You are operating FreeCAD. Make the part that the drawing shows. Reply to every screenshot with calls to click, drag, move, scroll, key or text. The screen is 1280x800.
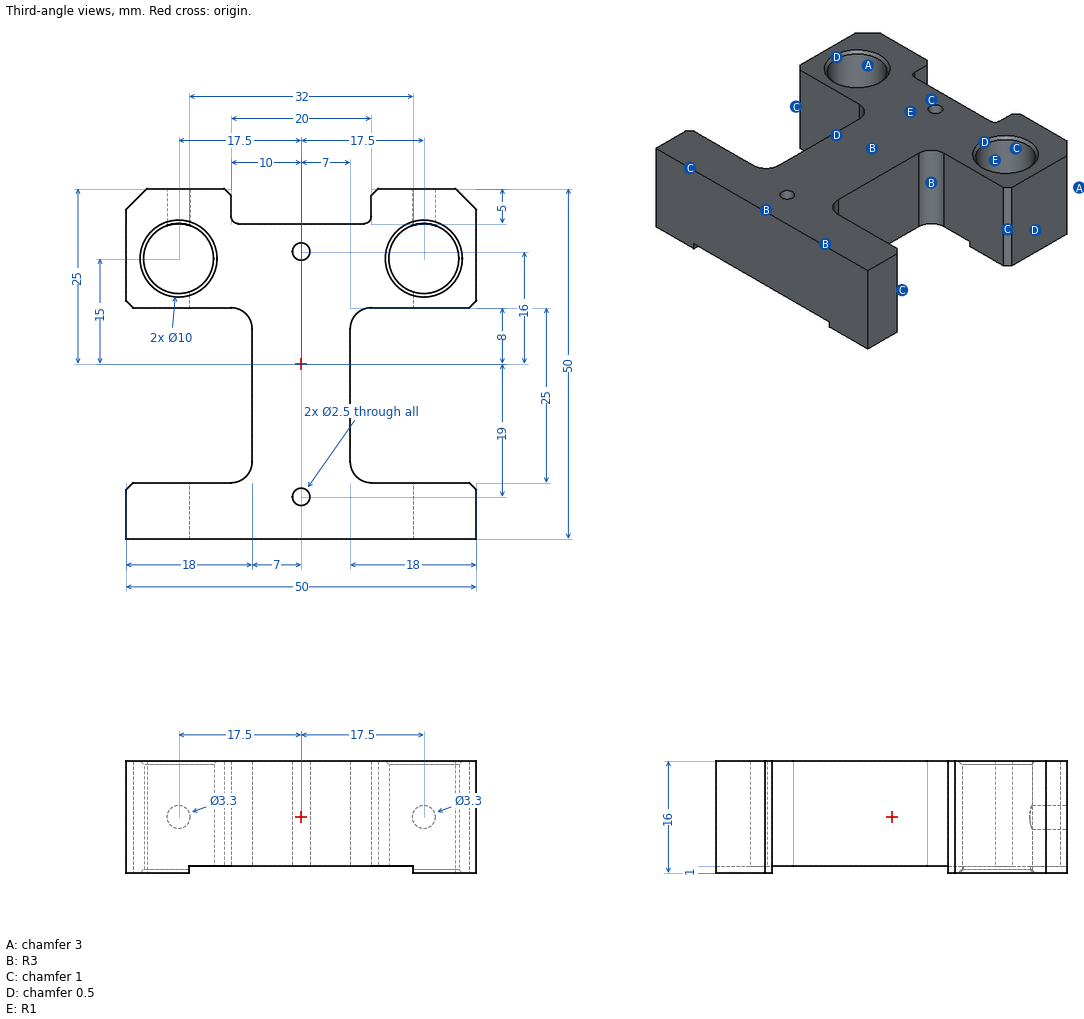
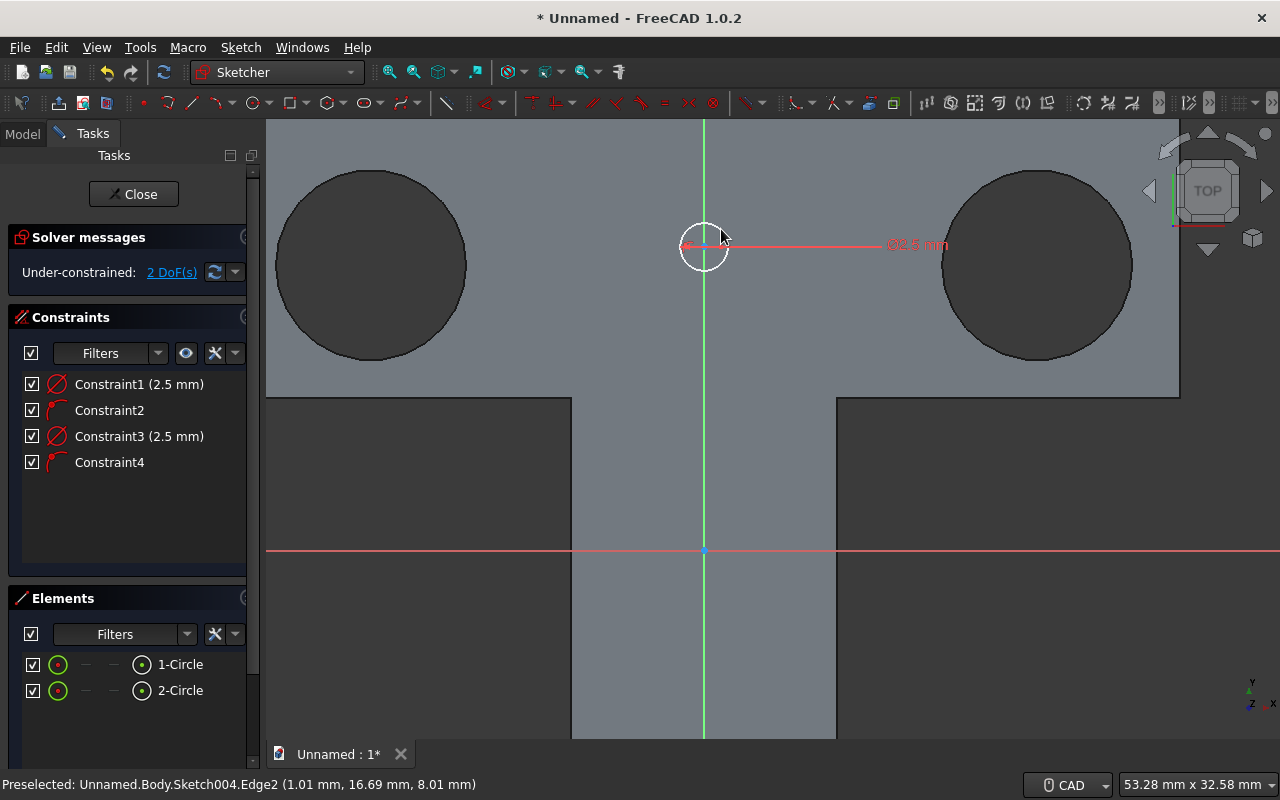
key(d)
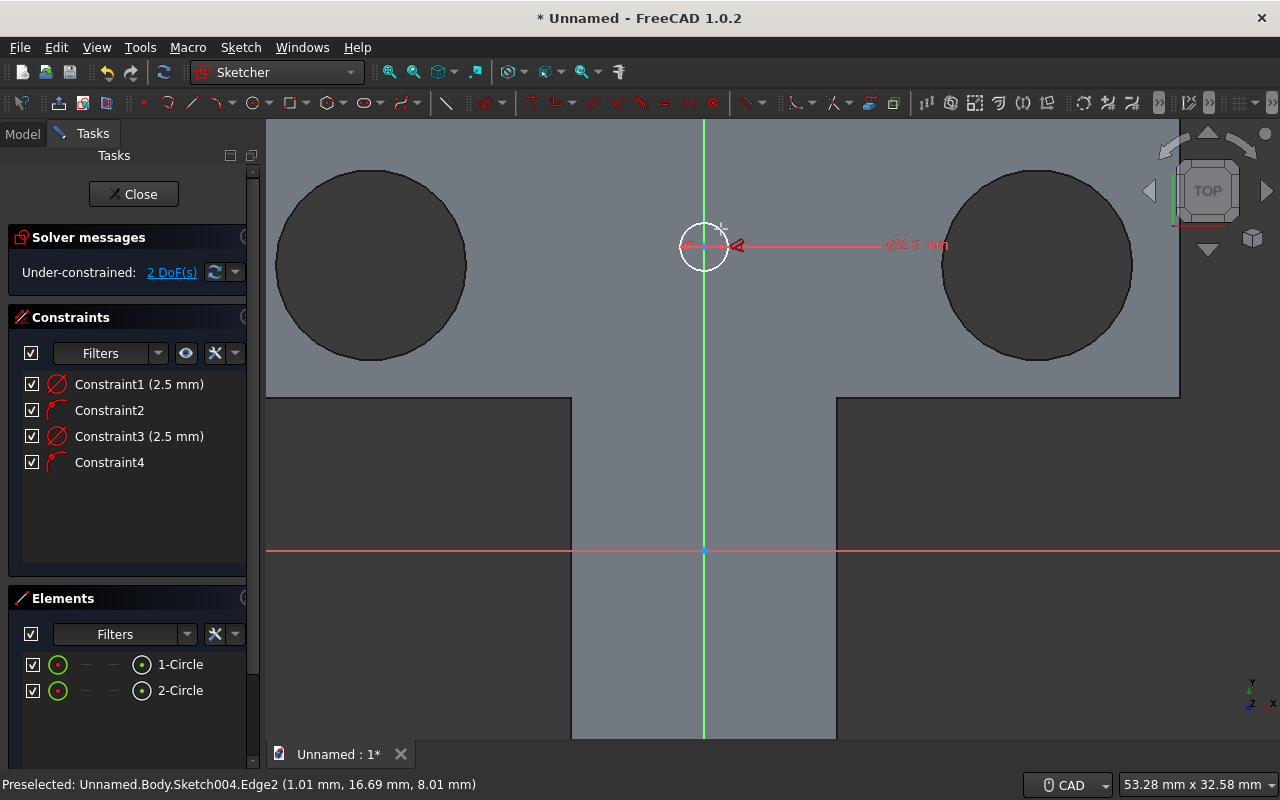
scroll(705, 246, down, 3)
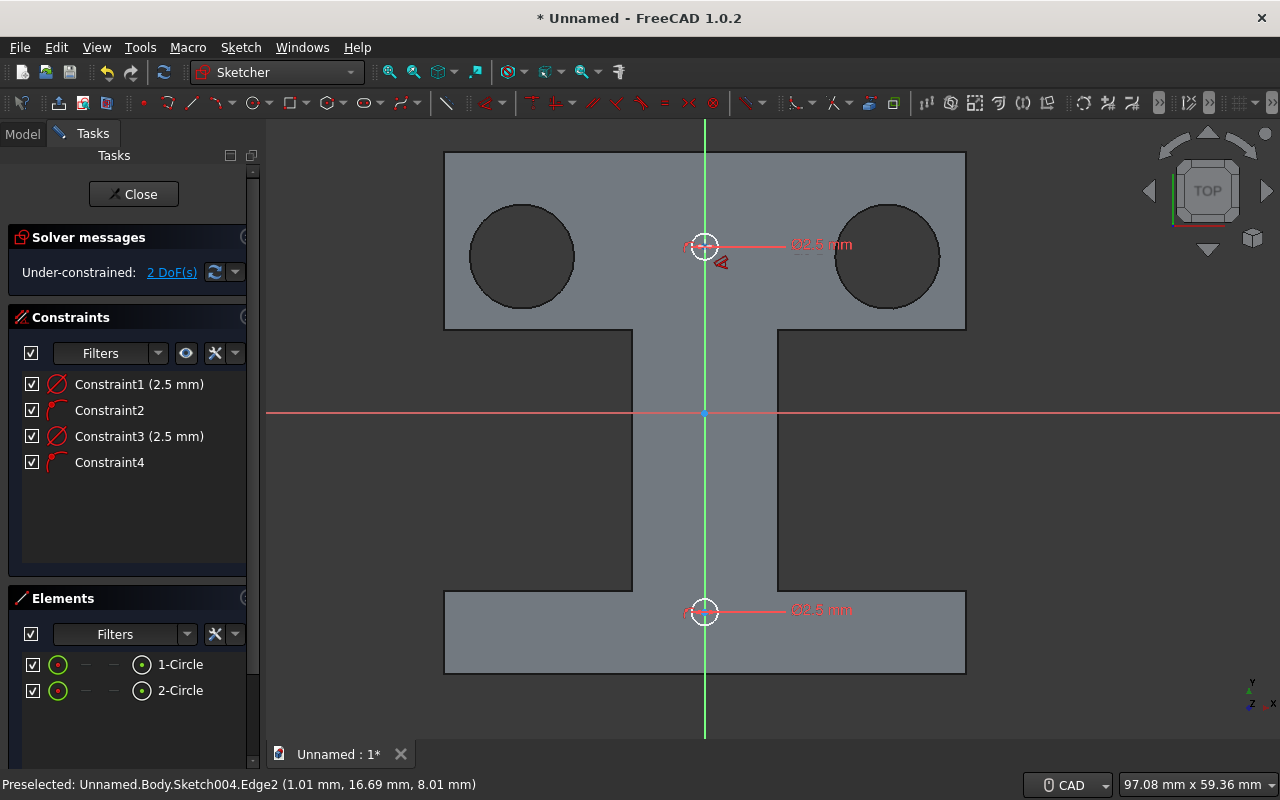
click(705, 612)
click(739, 513)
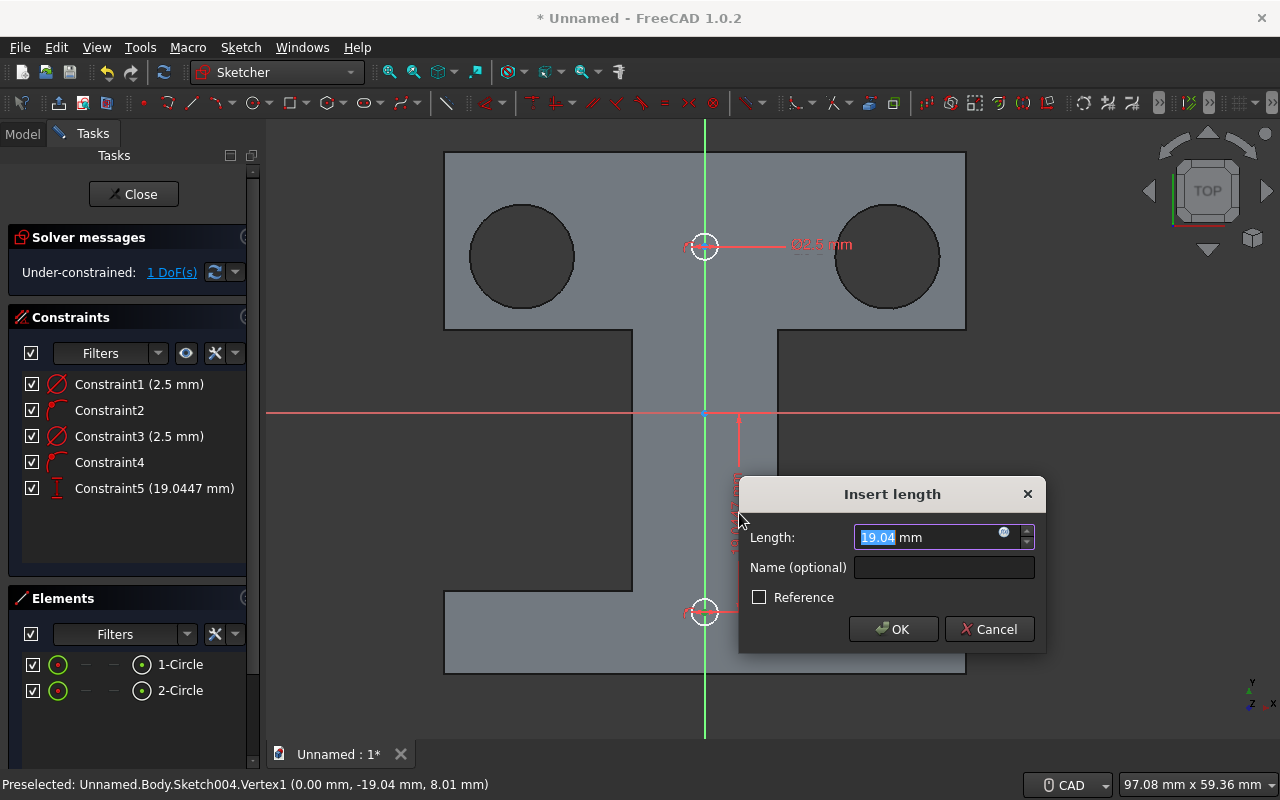
text(19)
key(Return)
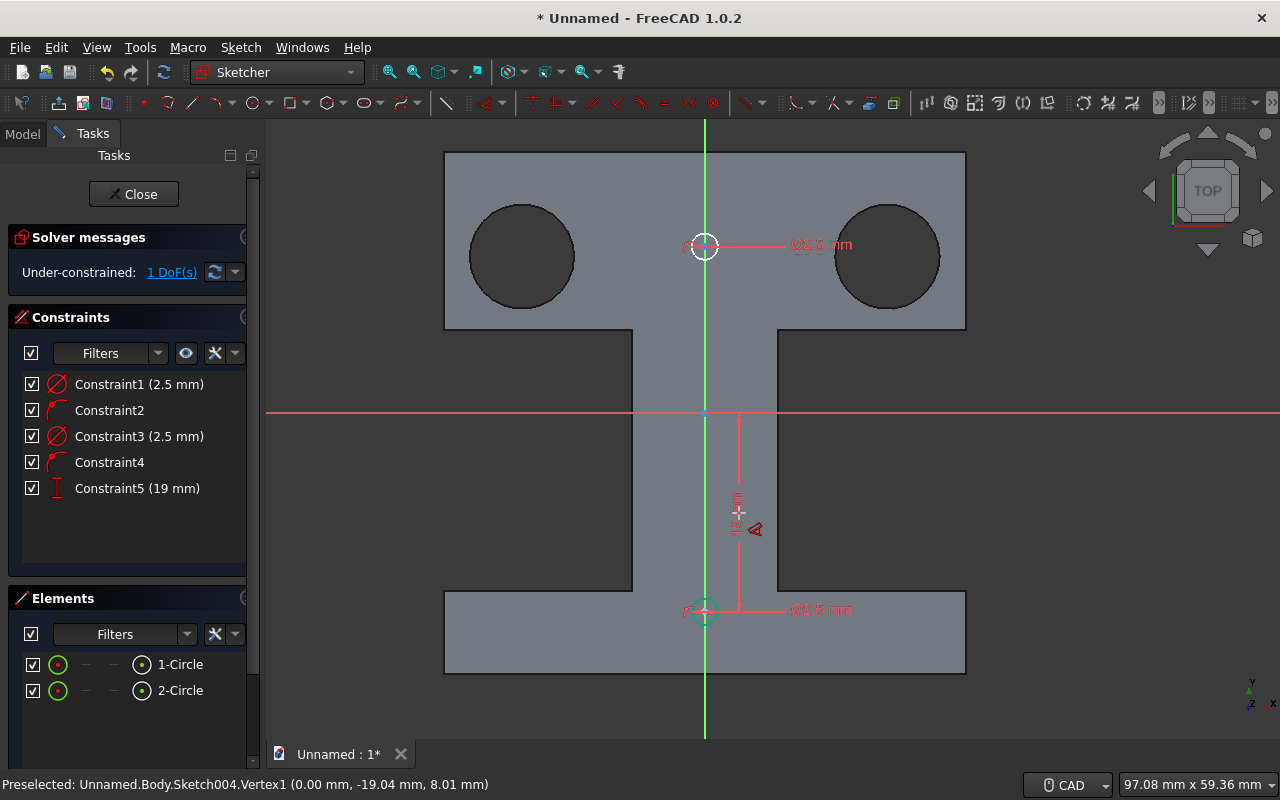
click(705, 247)
click(739, 330)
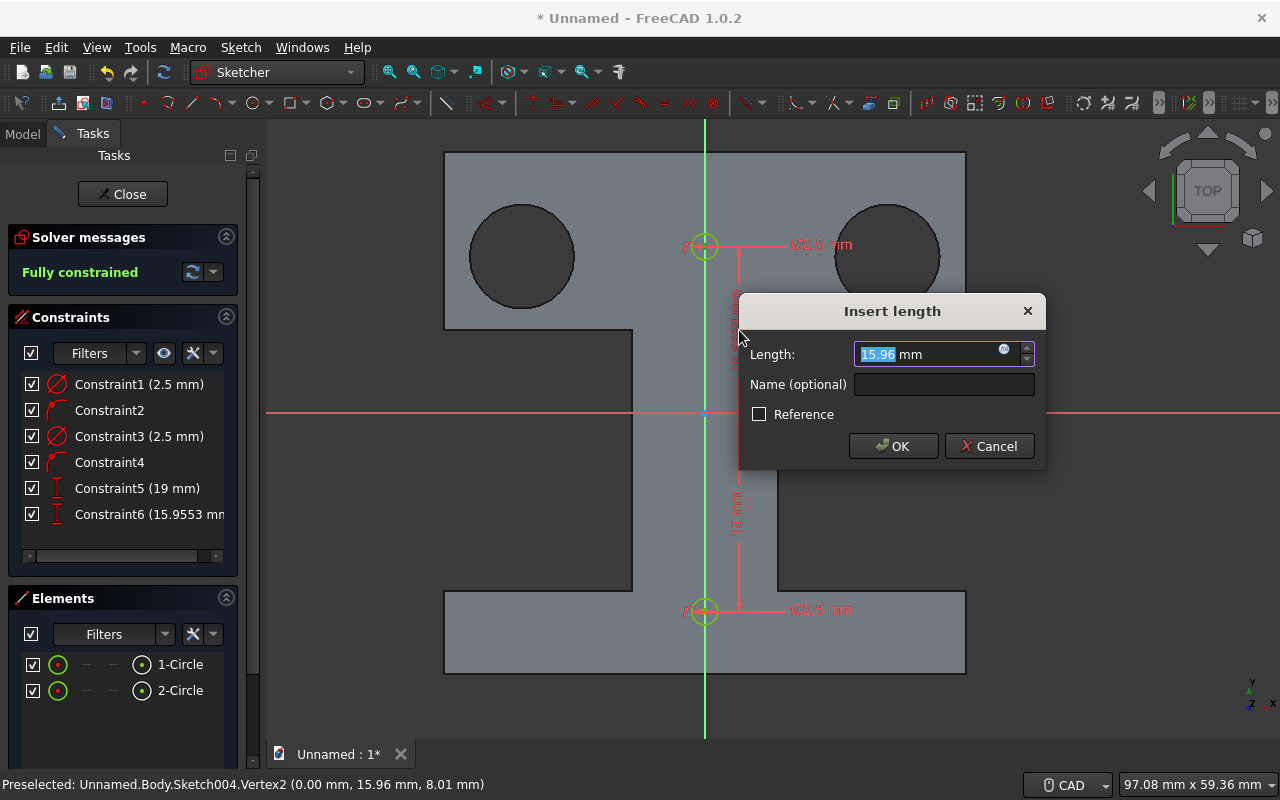
text(16)
key(Return)
key(Escape)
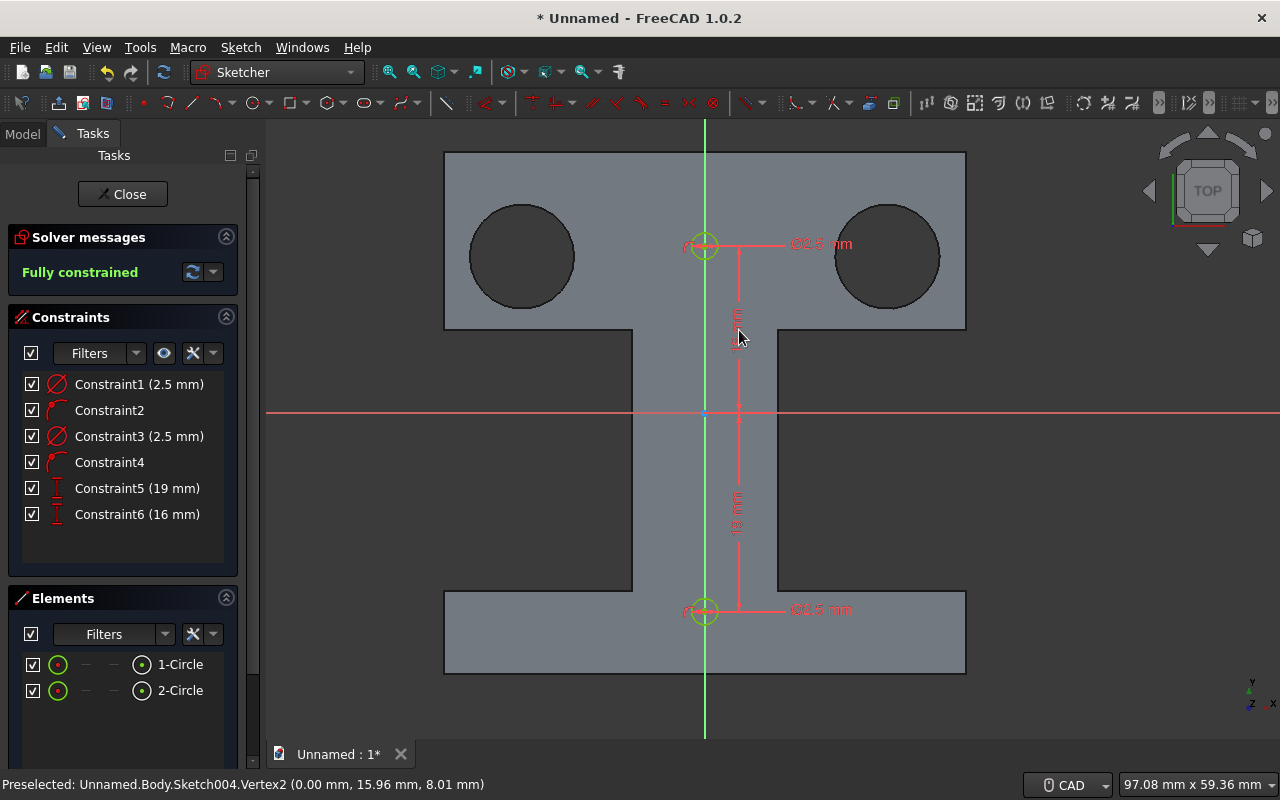
click(123, 194)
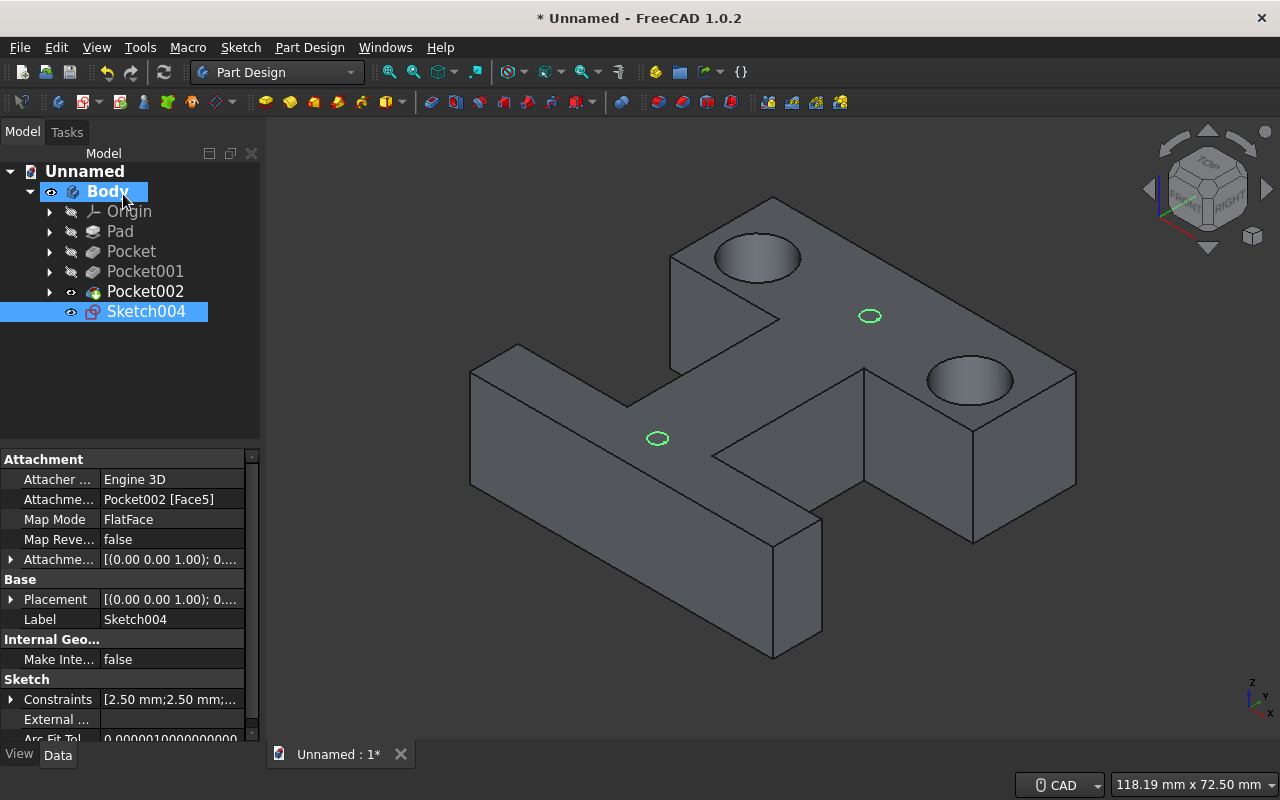
click(456, 102)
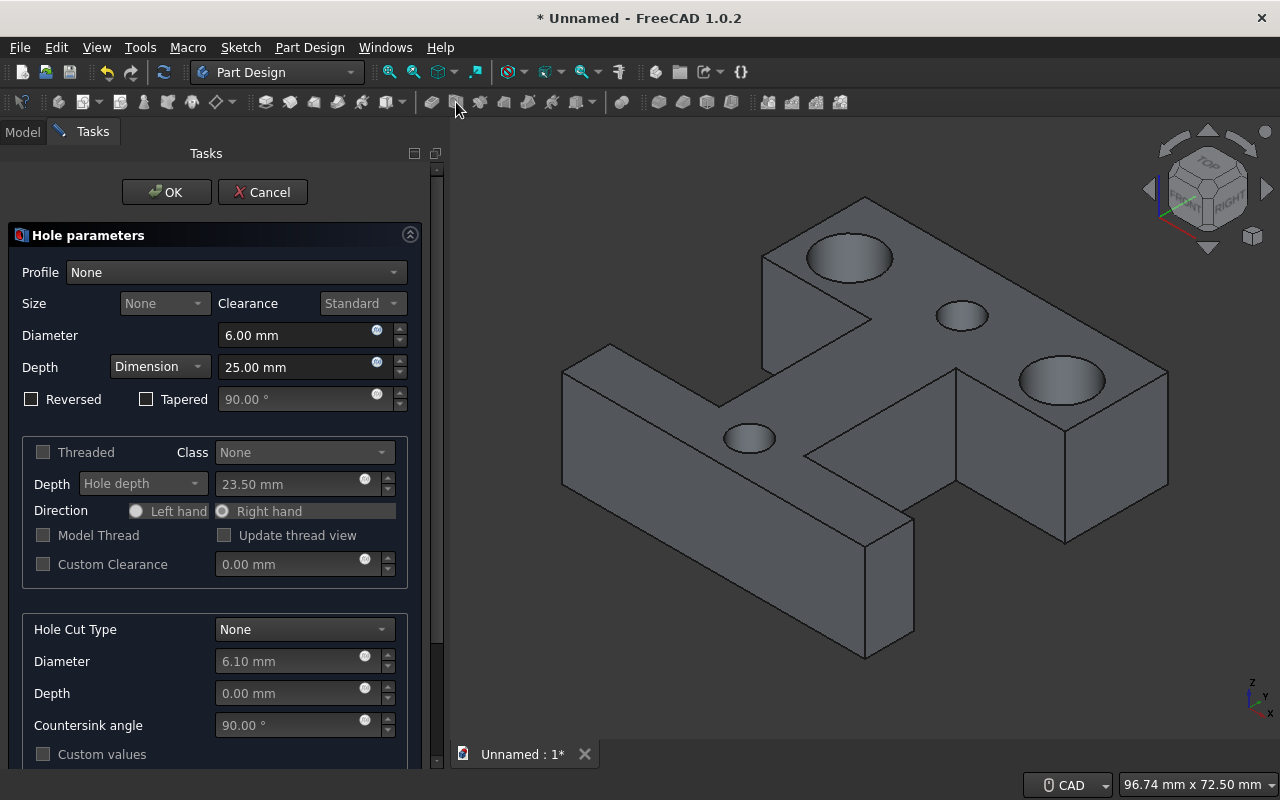
triple_click(305, 335)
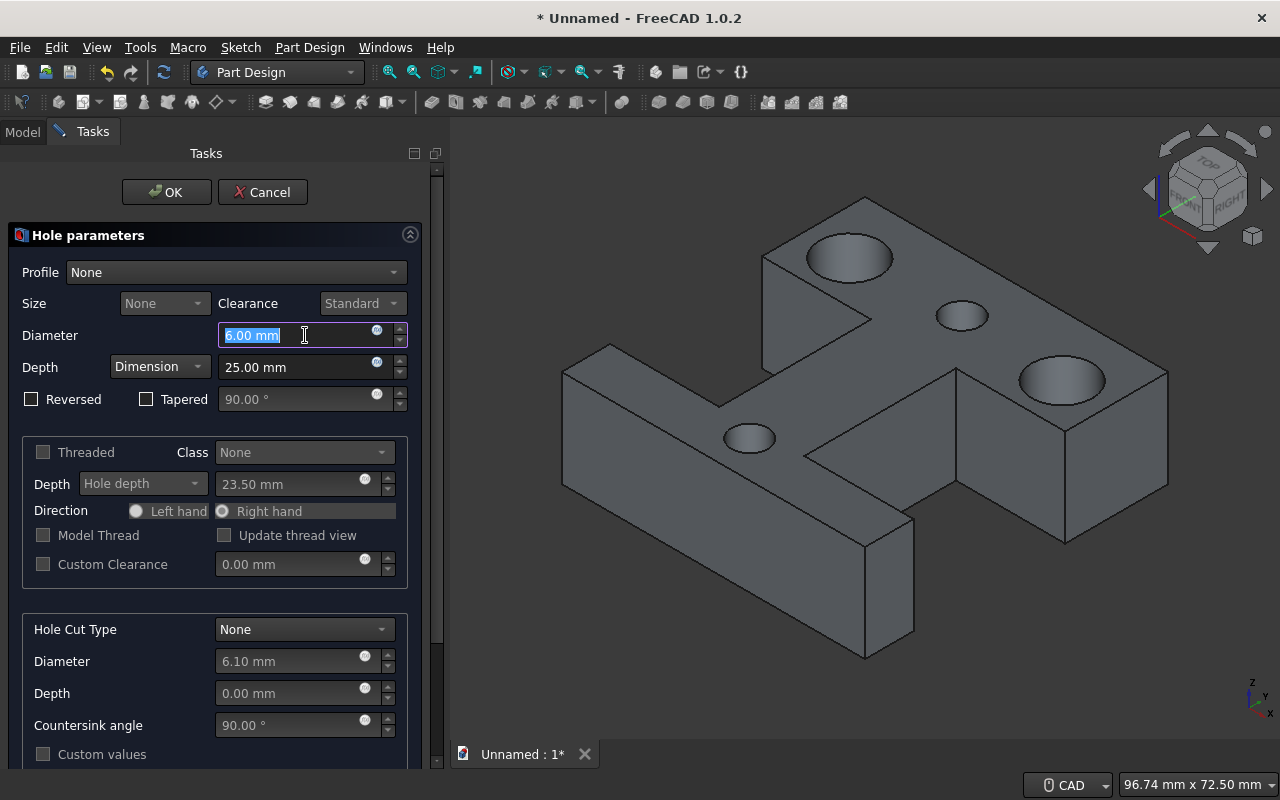
text(2.5)
key(Tab)